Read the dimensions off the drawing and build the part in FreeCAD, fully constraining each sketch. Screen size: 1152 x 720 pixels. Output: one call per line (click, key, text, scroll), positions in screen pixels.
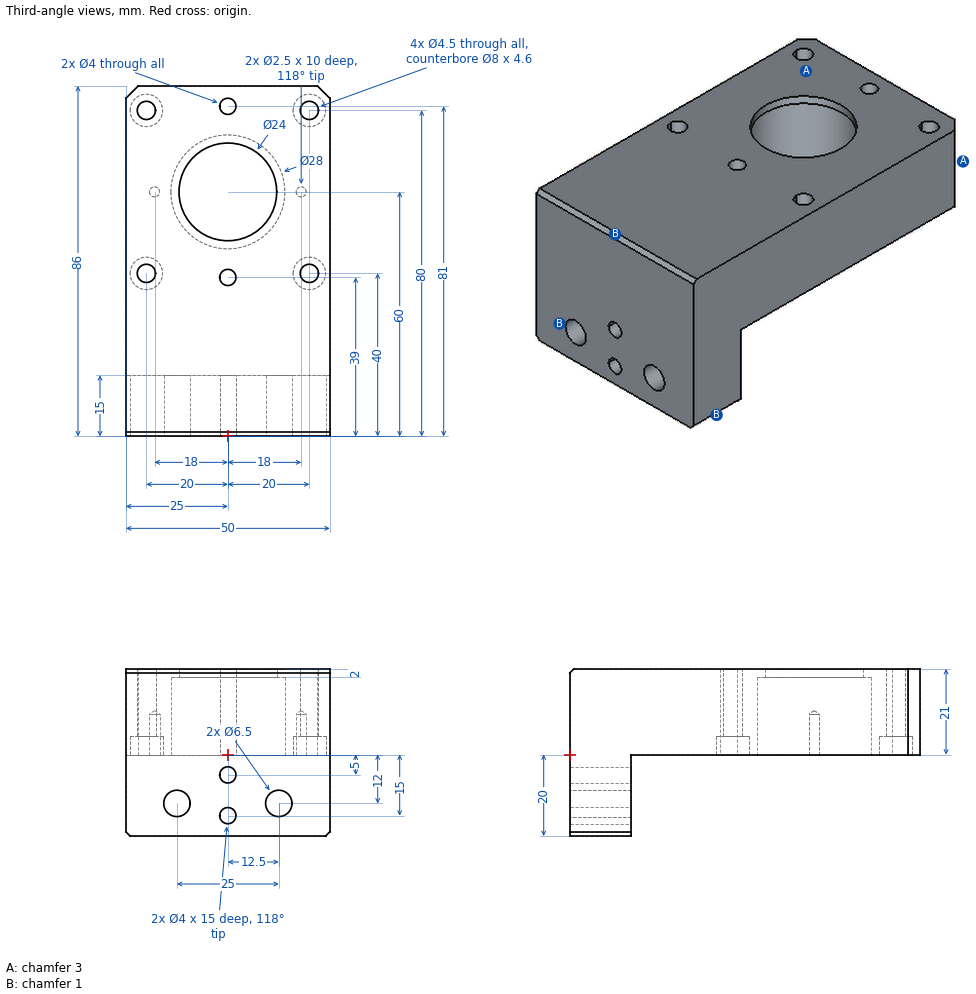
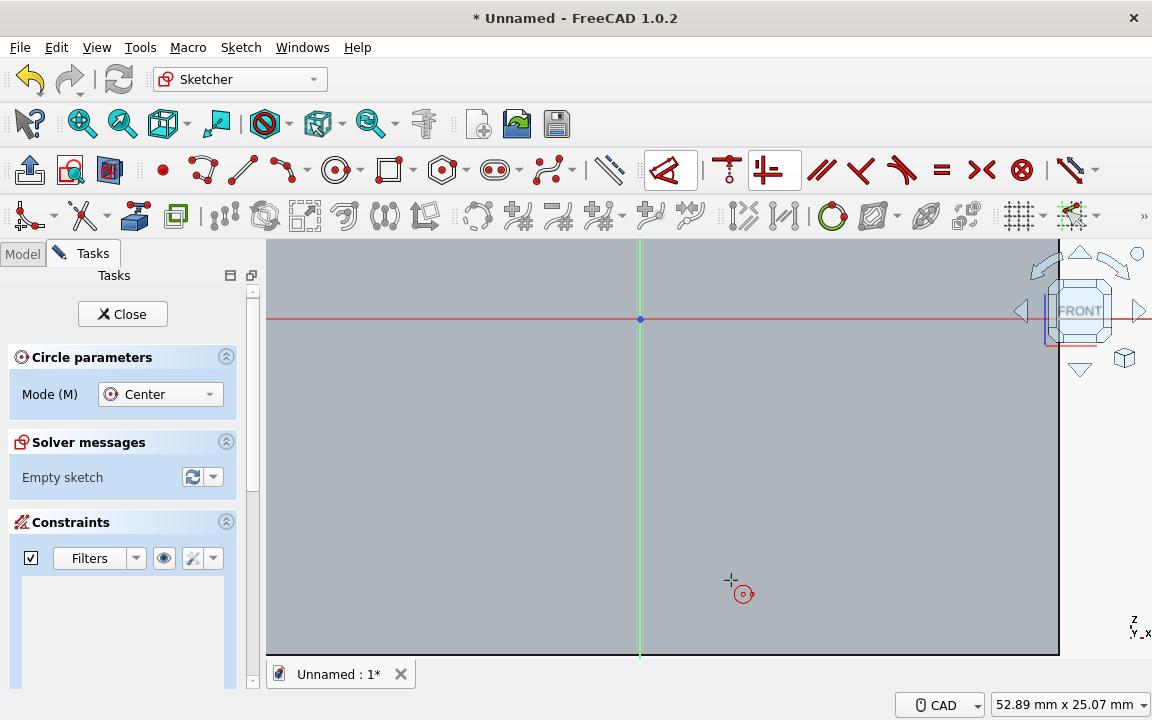
click(850, 520)
click(888, 482)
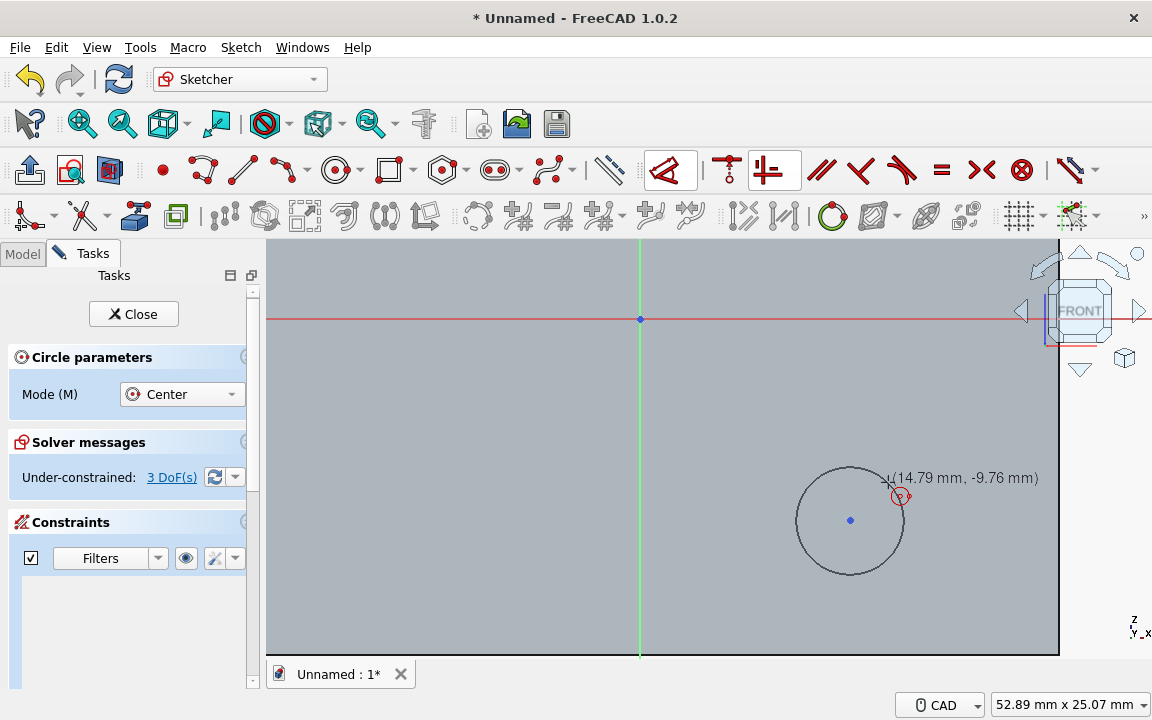
click(431, 520)
click(469, 482)
key(Escape)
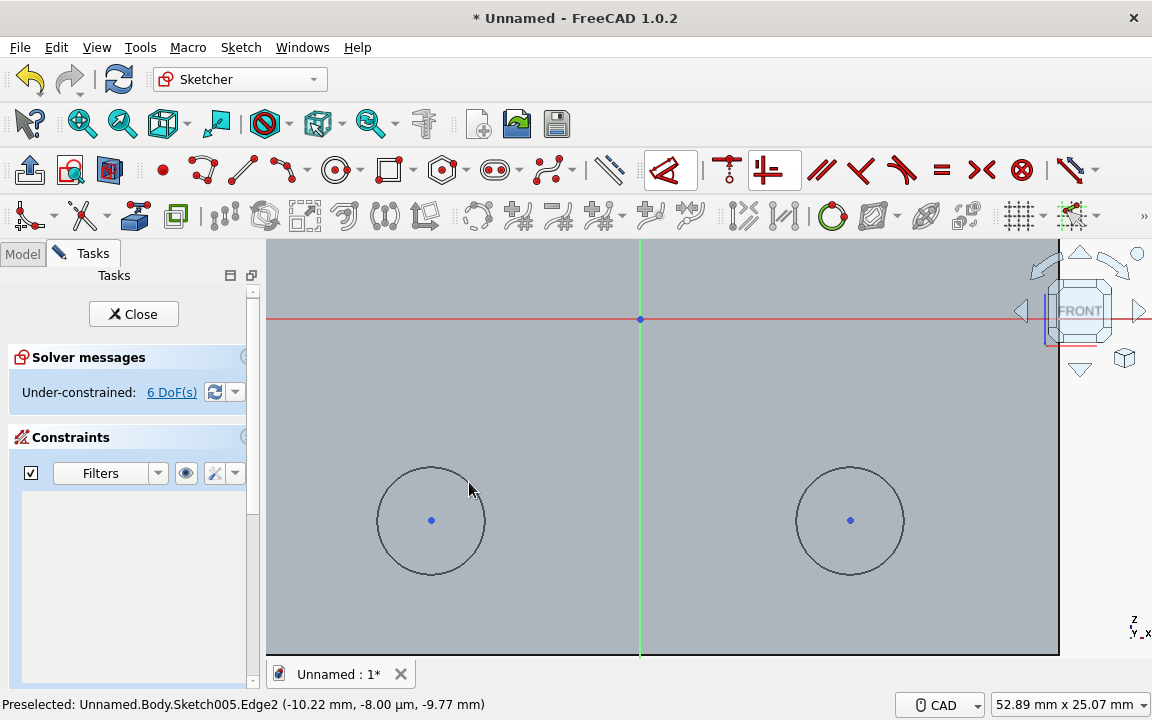
click(888, 483)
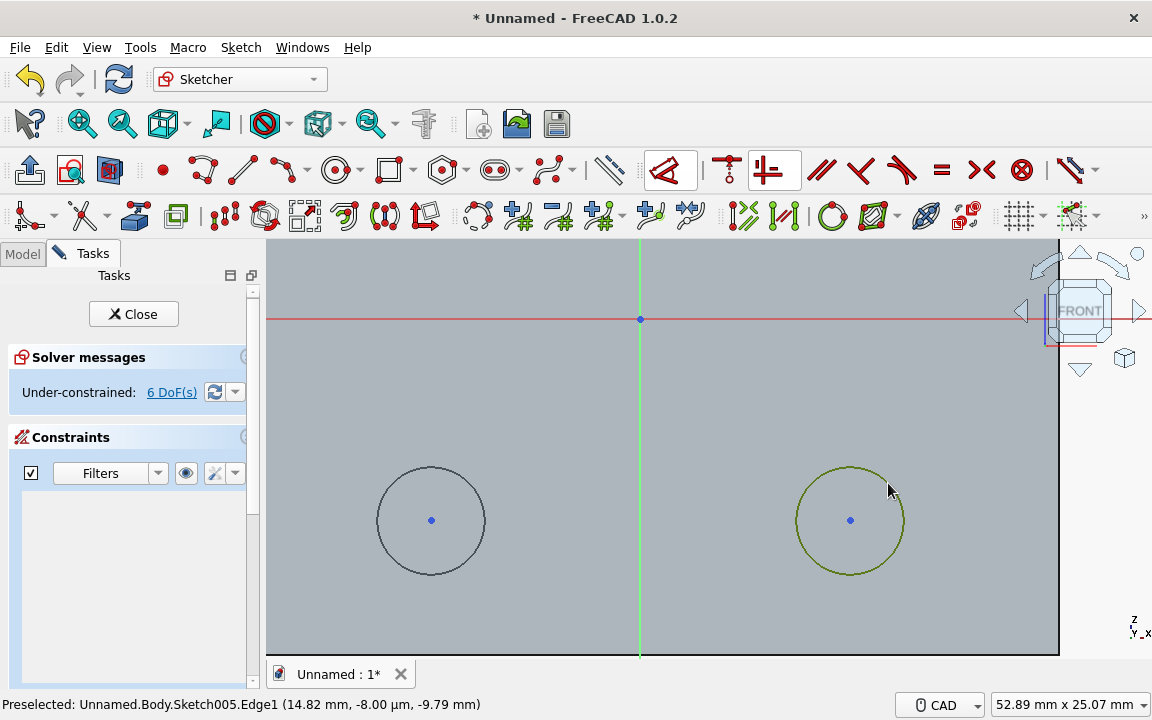
click(469, 483)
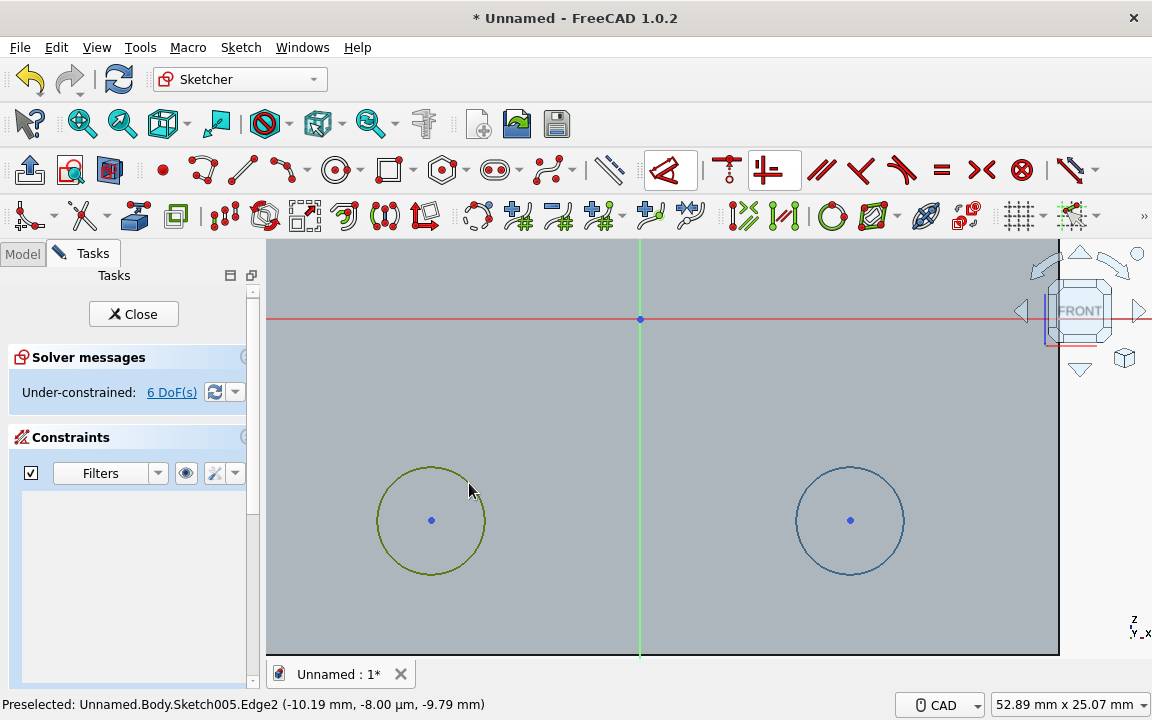
key(e)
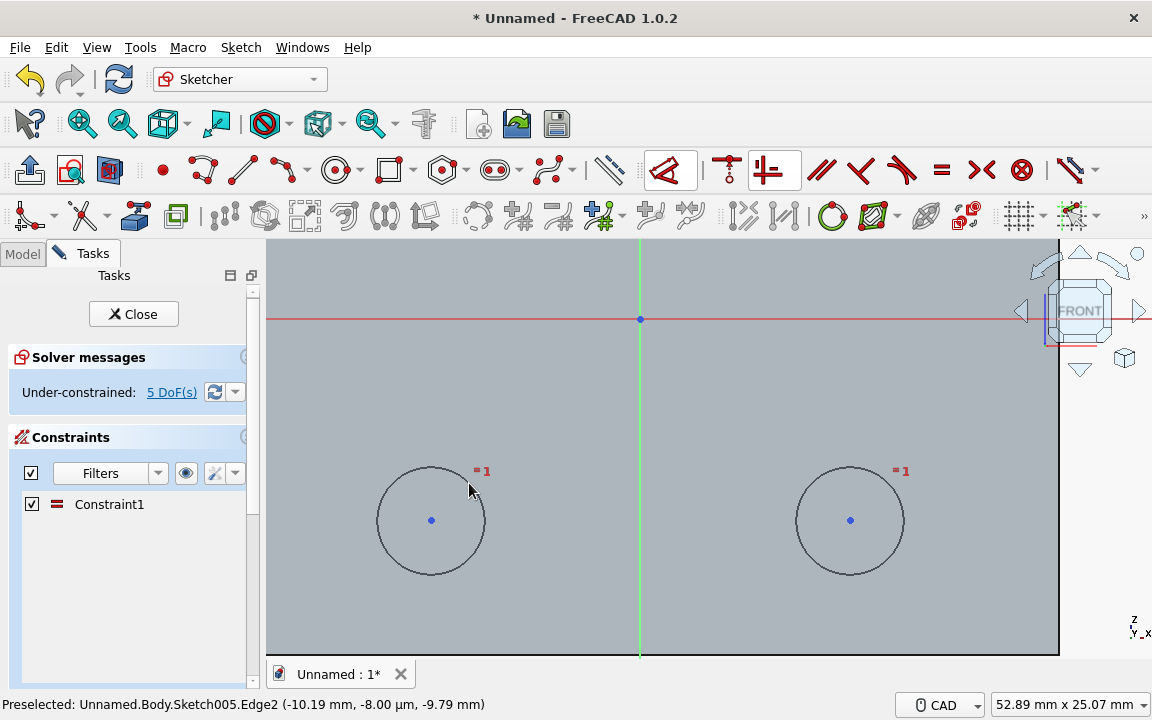
click(850, 521)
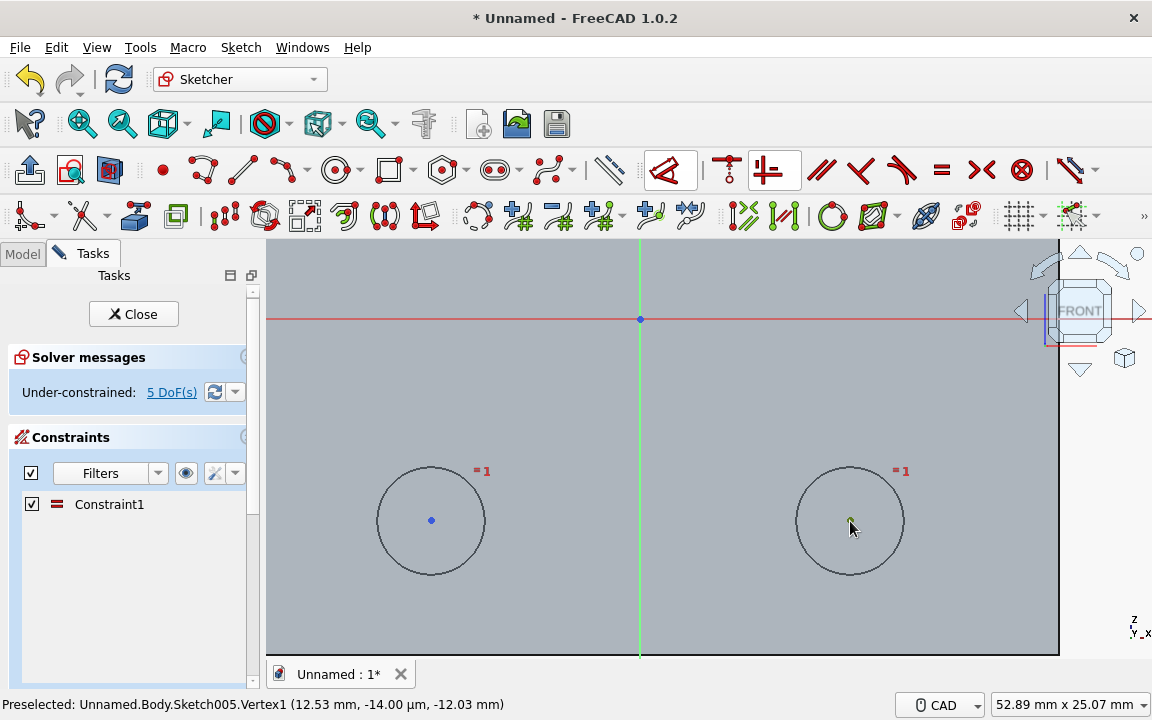
click(431, 521)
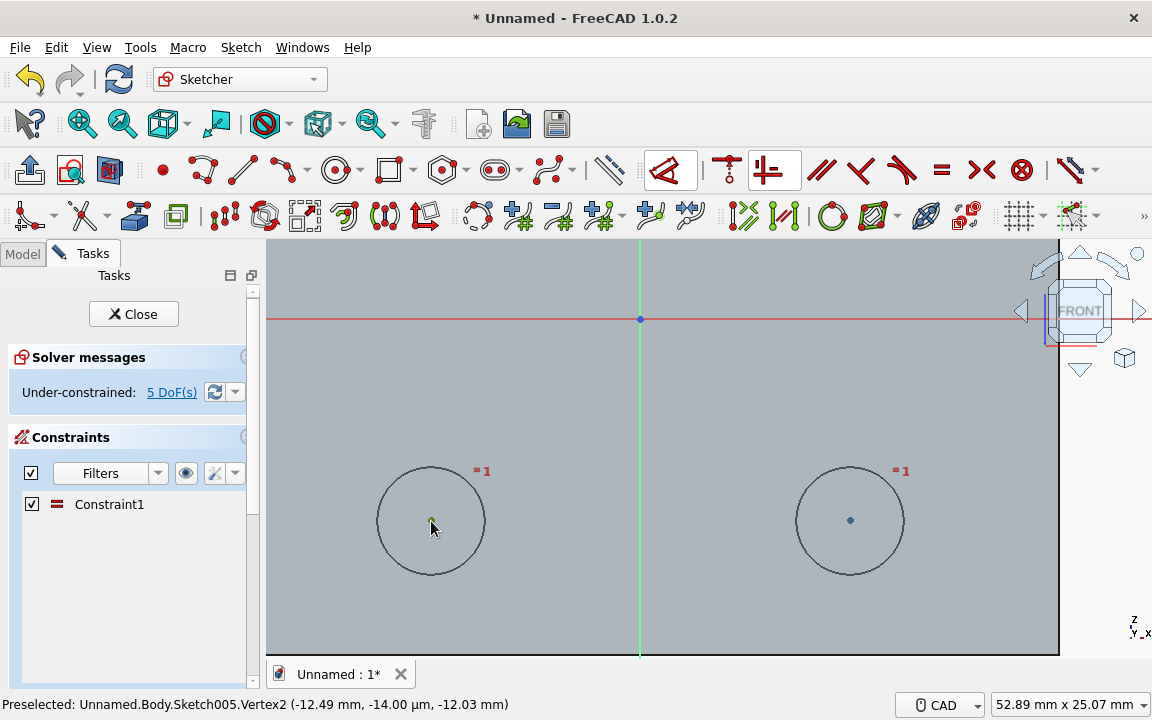
click(796, 170)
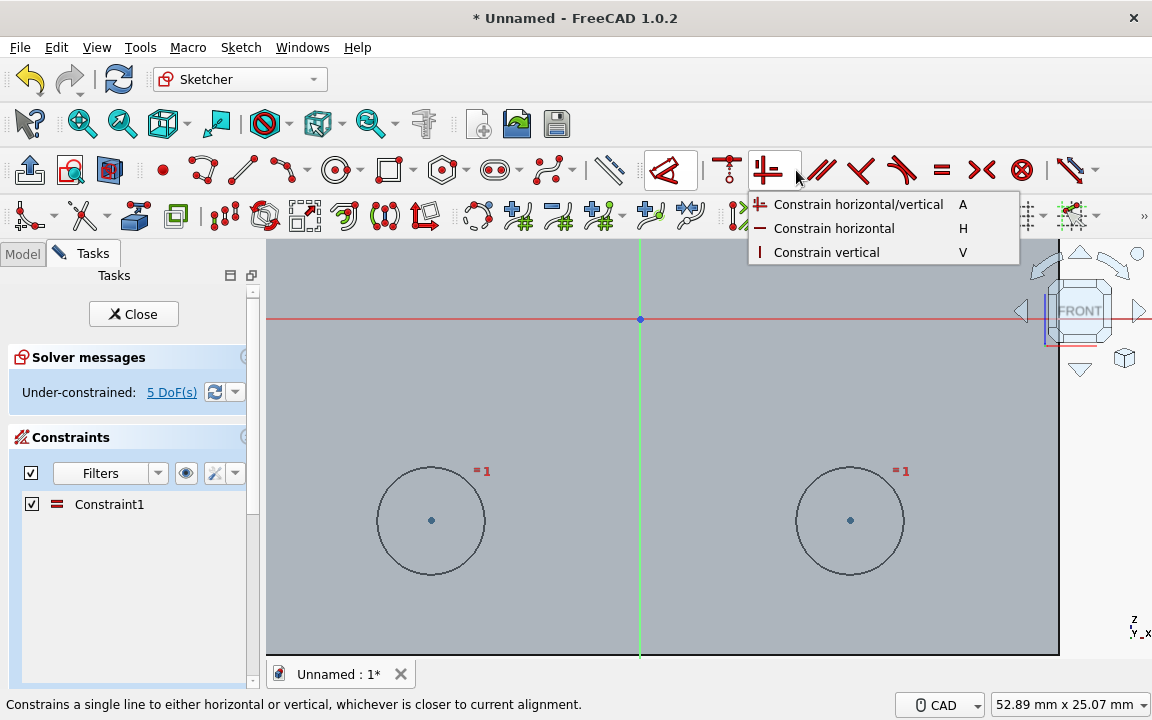
click(884, 228)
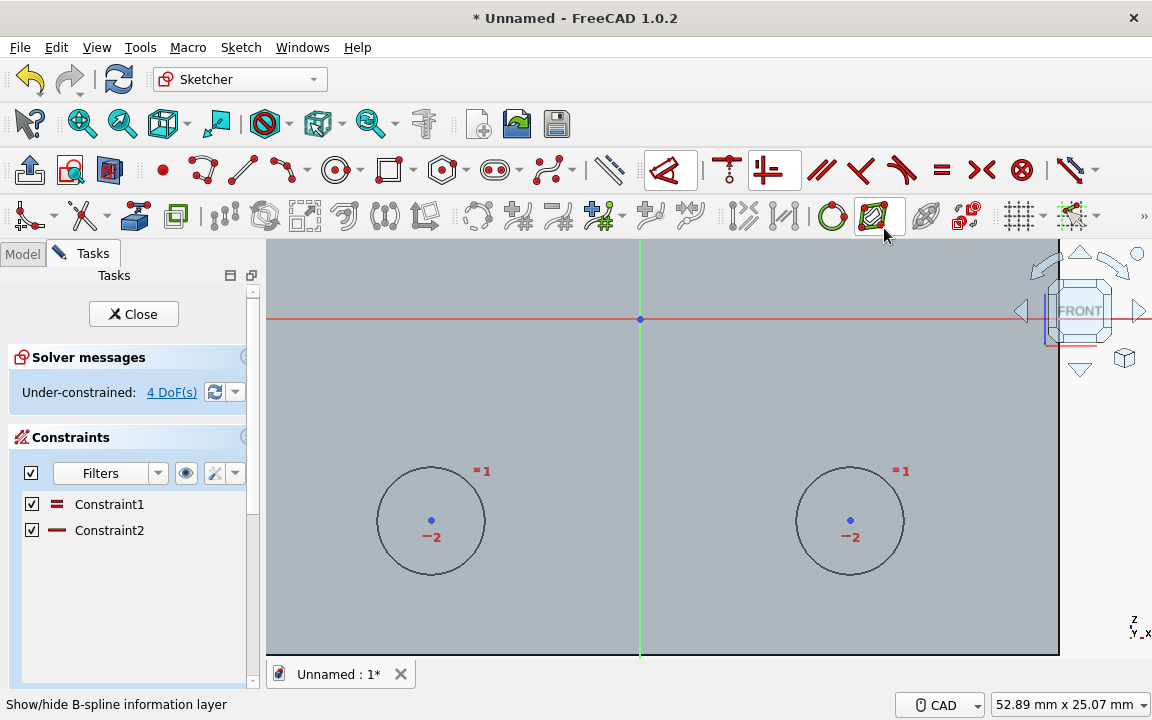
click(888, 483)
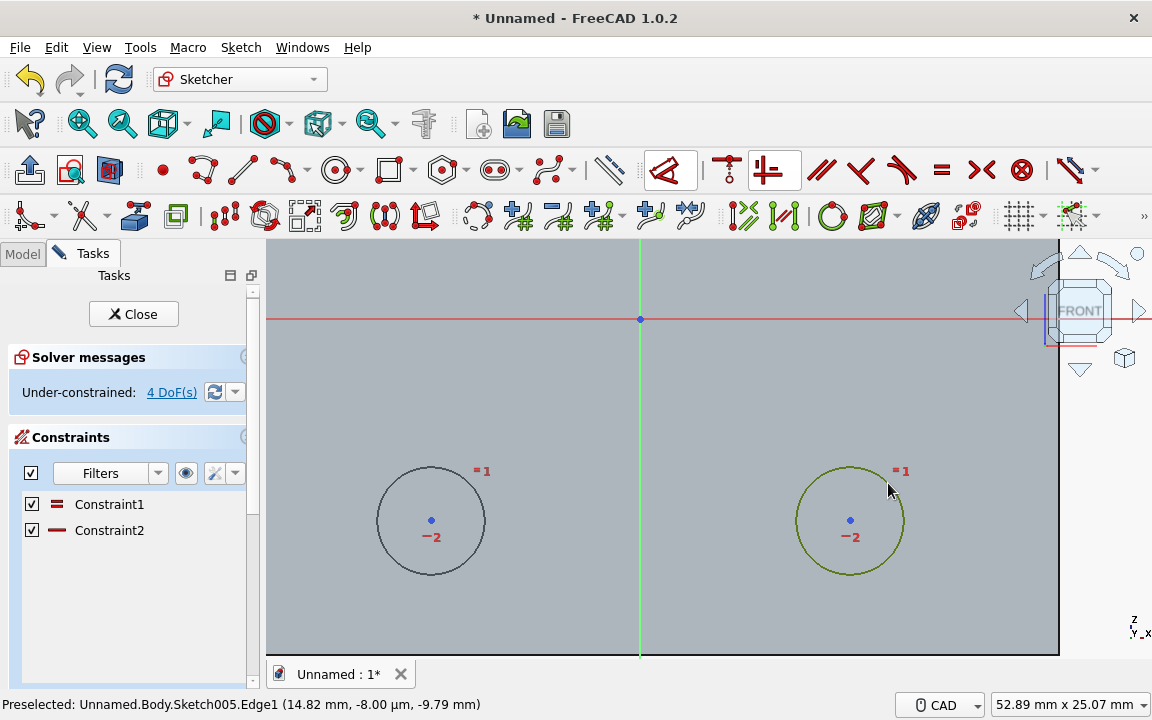
click(692, 170)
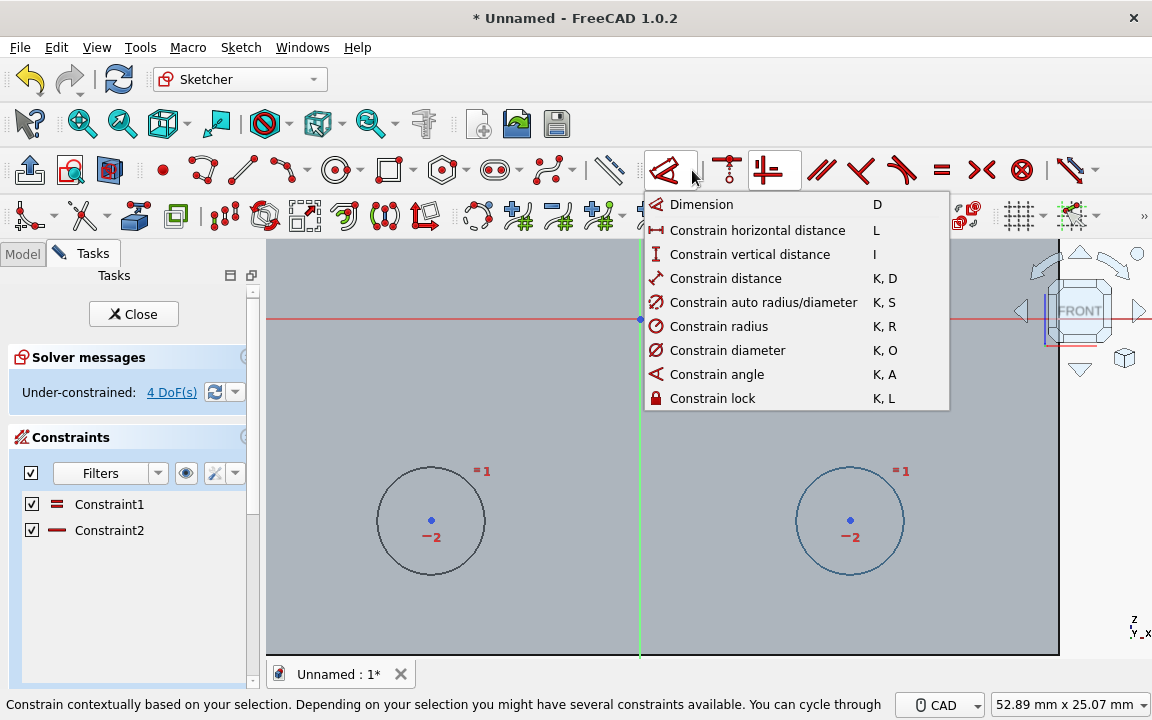
click(797, 350)